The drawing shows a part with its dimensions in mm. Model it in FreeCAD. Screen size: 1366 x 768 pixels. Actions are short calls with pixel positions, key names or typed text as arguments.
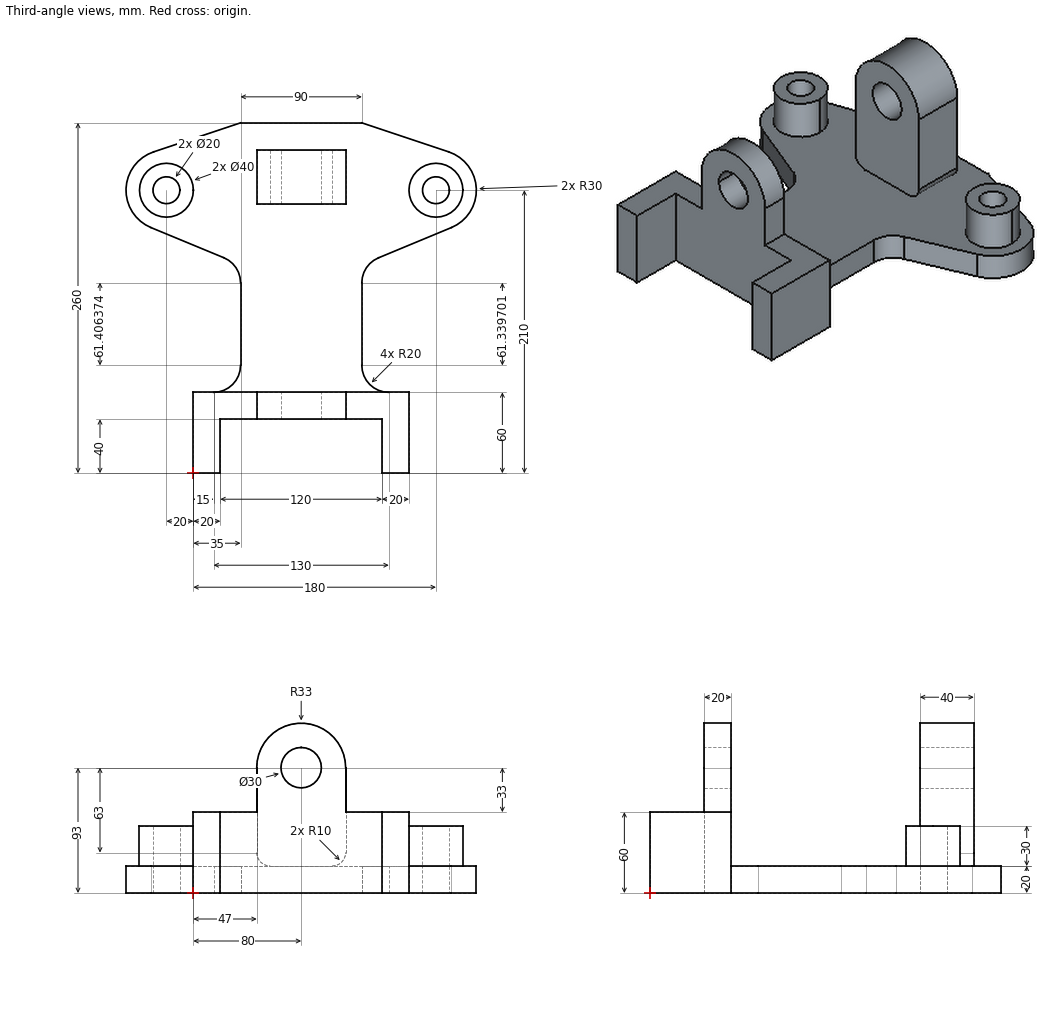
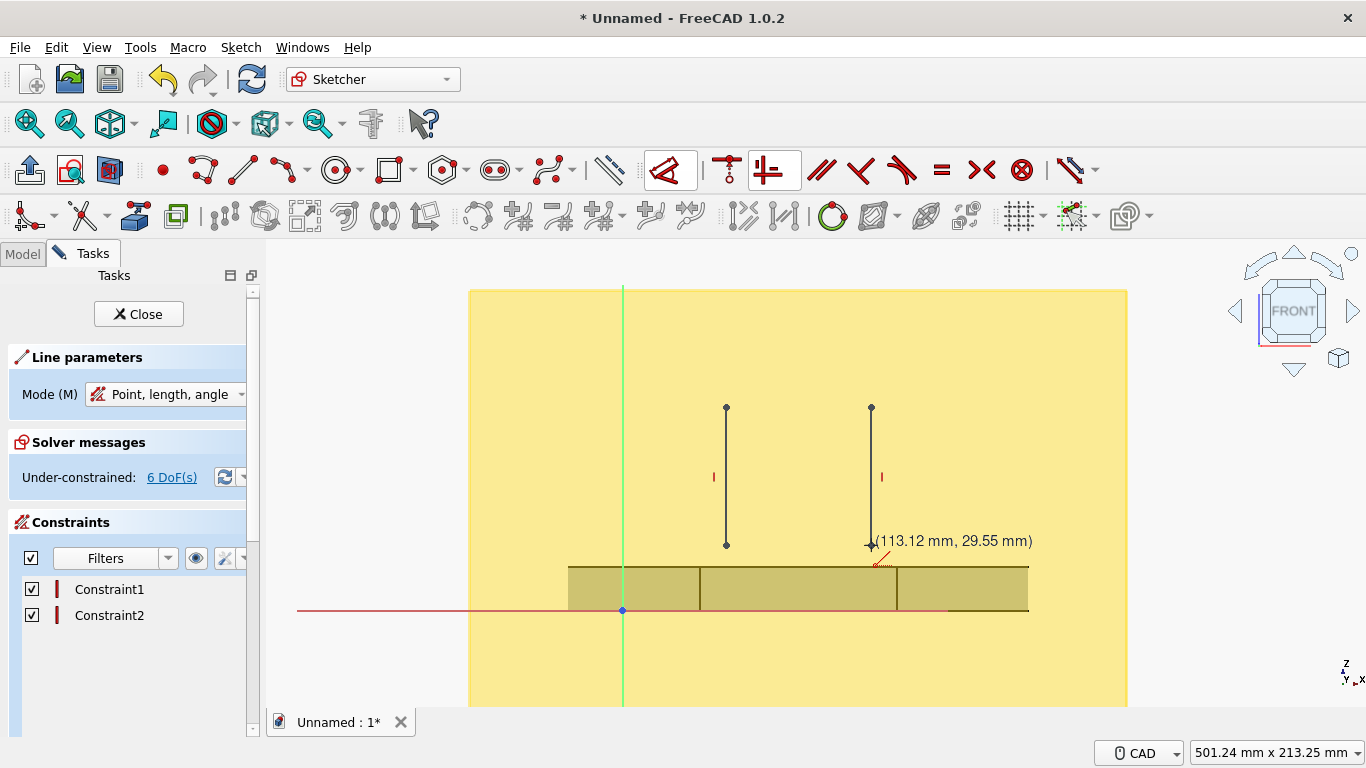
click(849, 567)
click(748, 567)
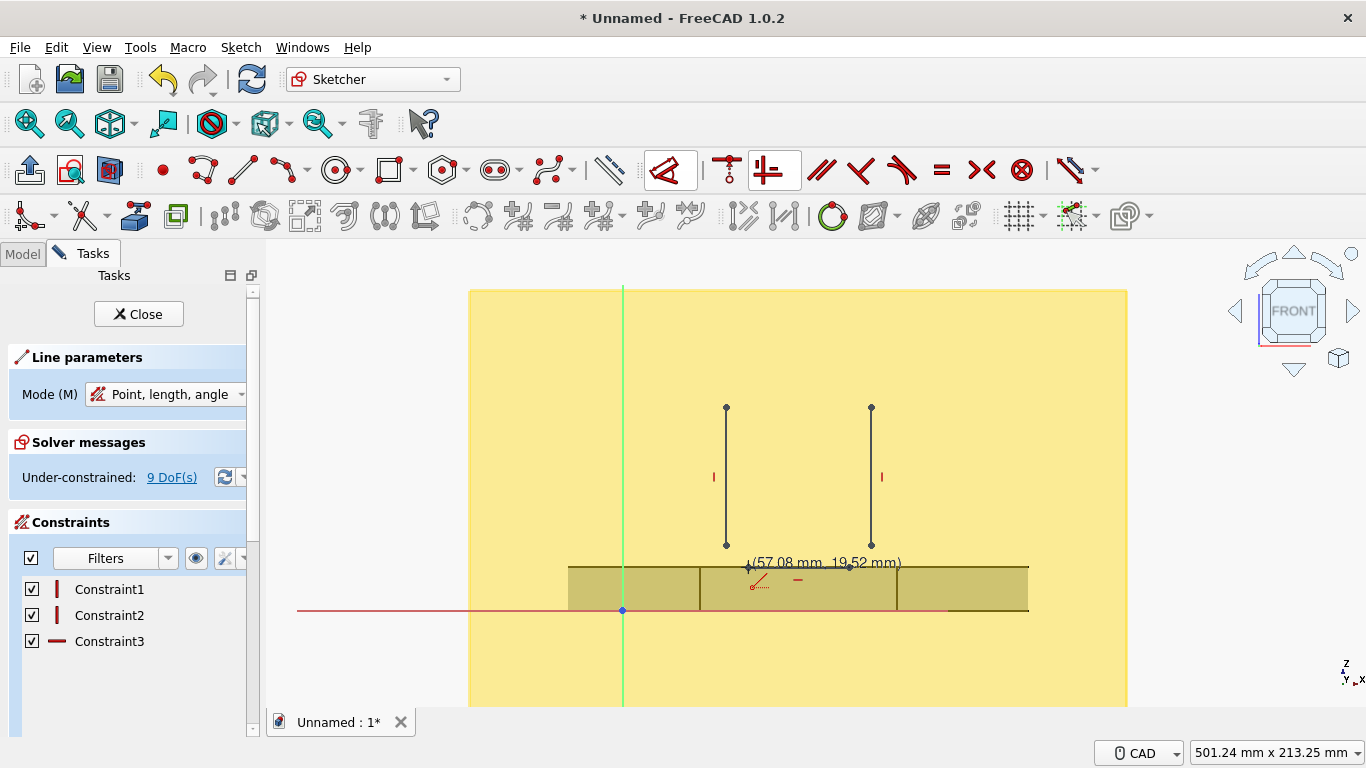
click(284, 170)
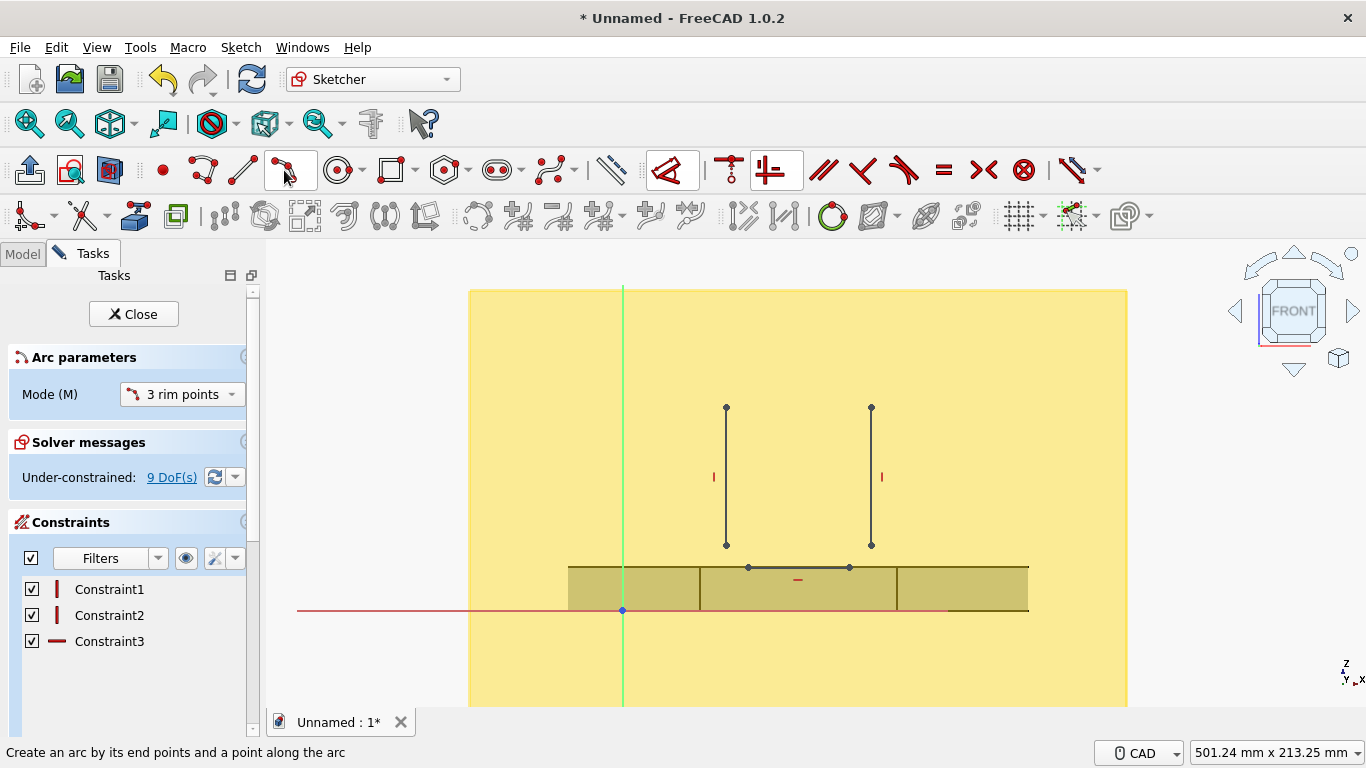
click(726, 408)
click(871, 408)
click(798, 334)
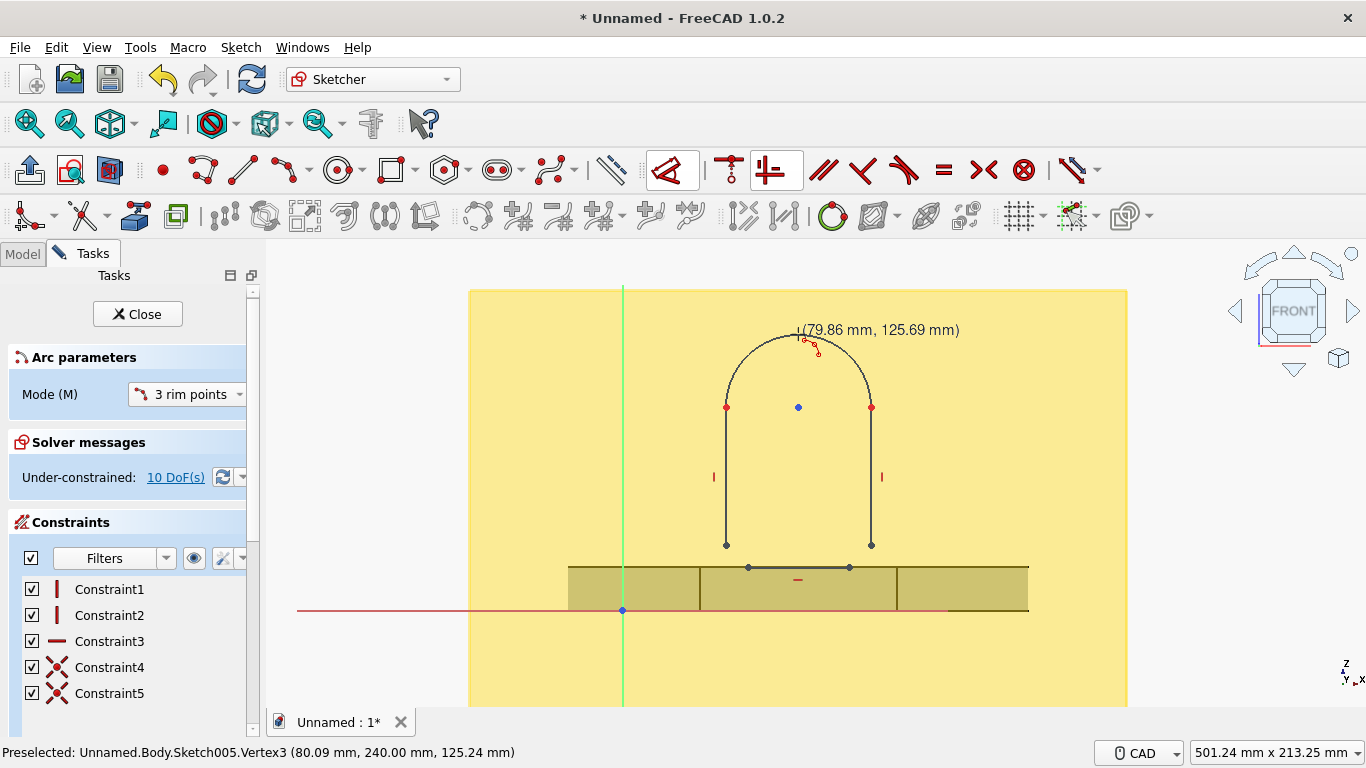
click(871, 546)
click(849, 568)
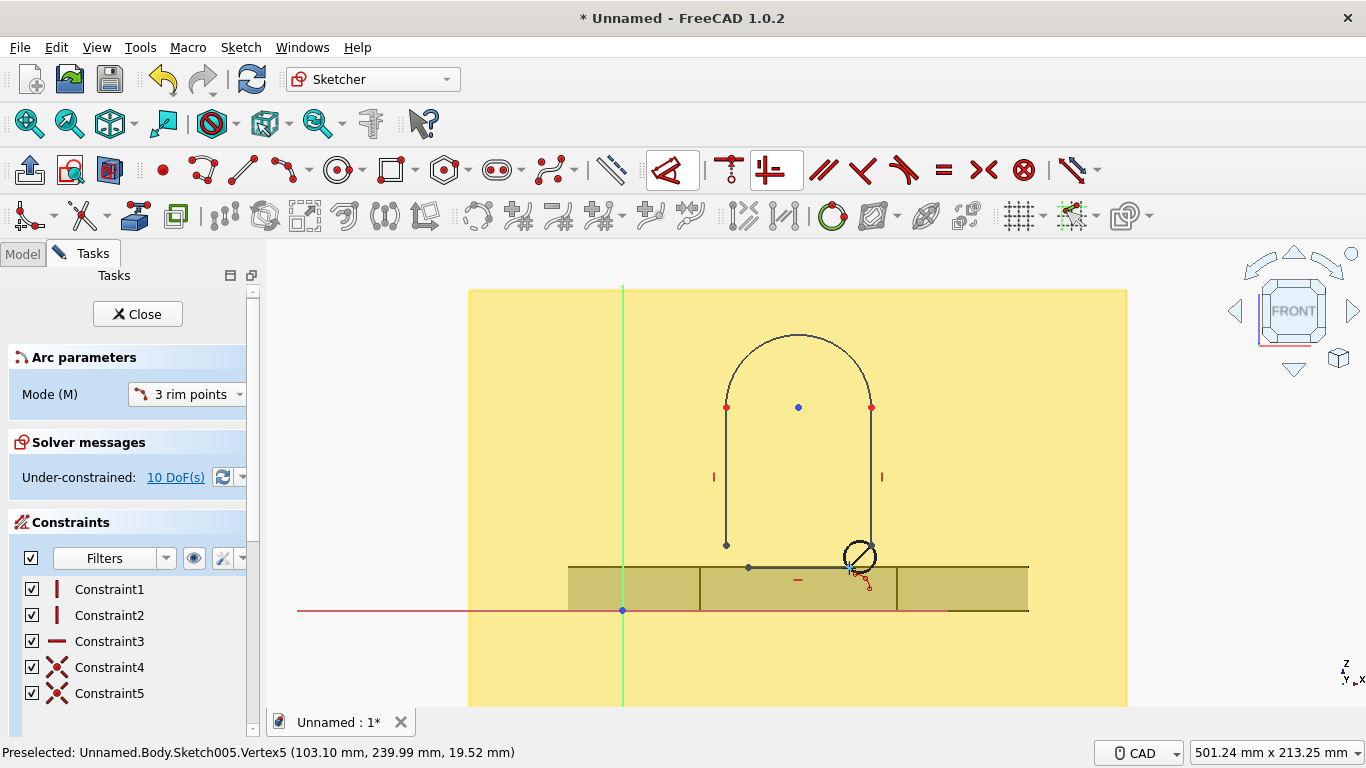
scroll(864, 561, up, 5)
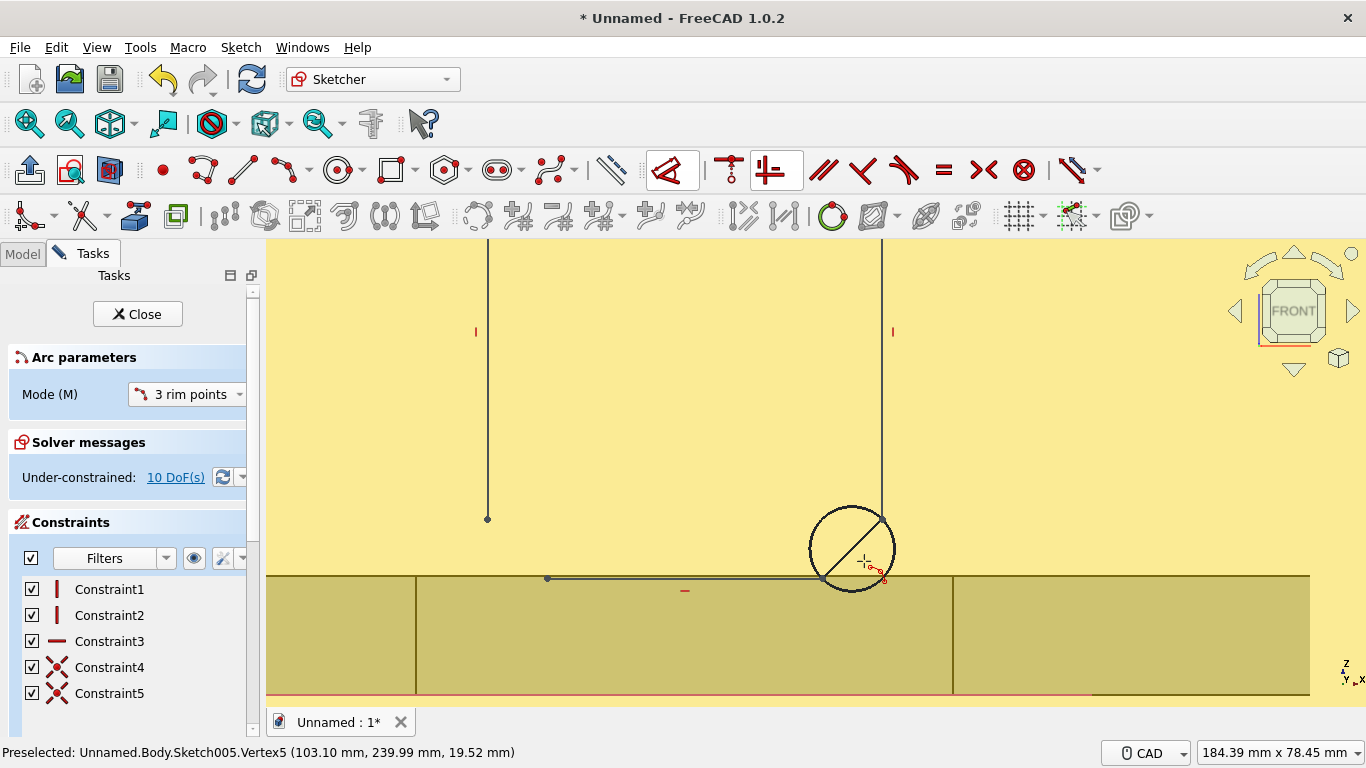
click(864, 559)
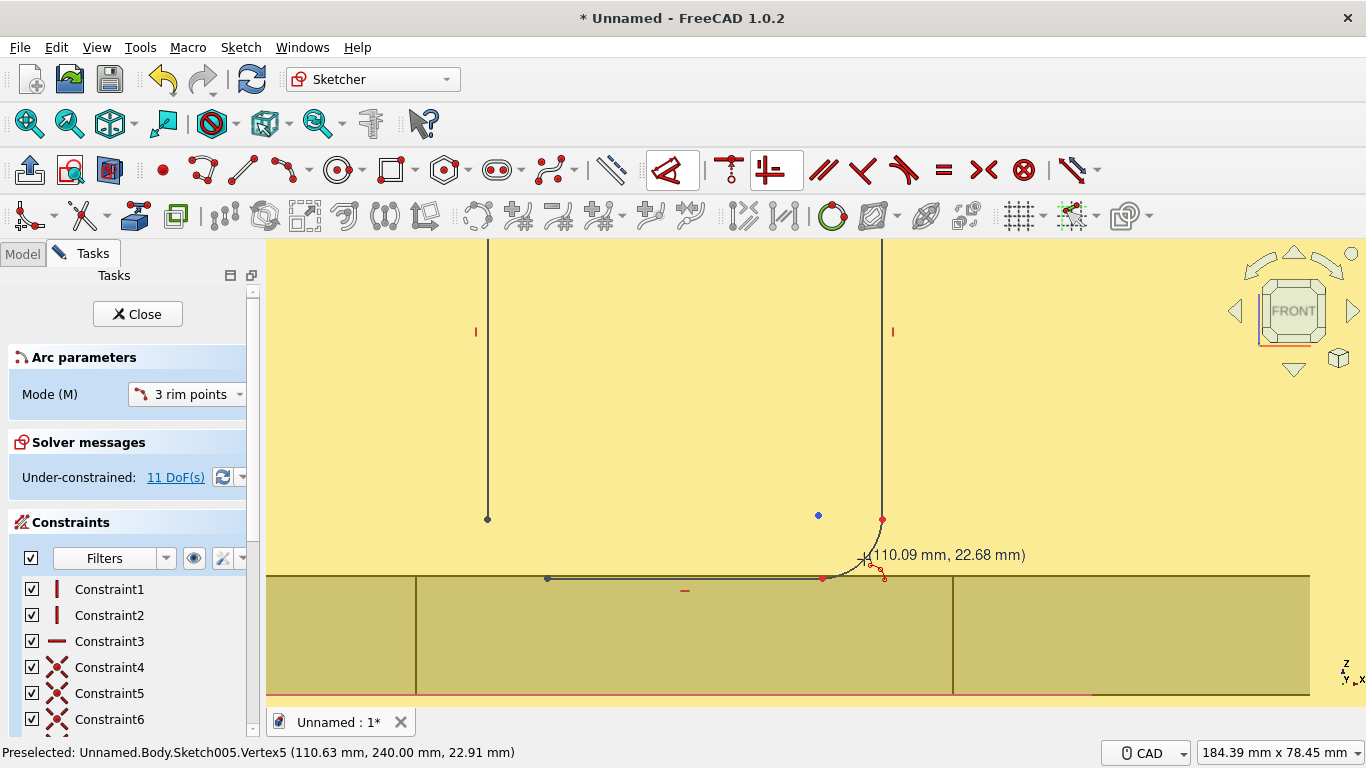
click(548, 579)
click(488, 519)
click(505, 559)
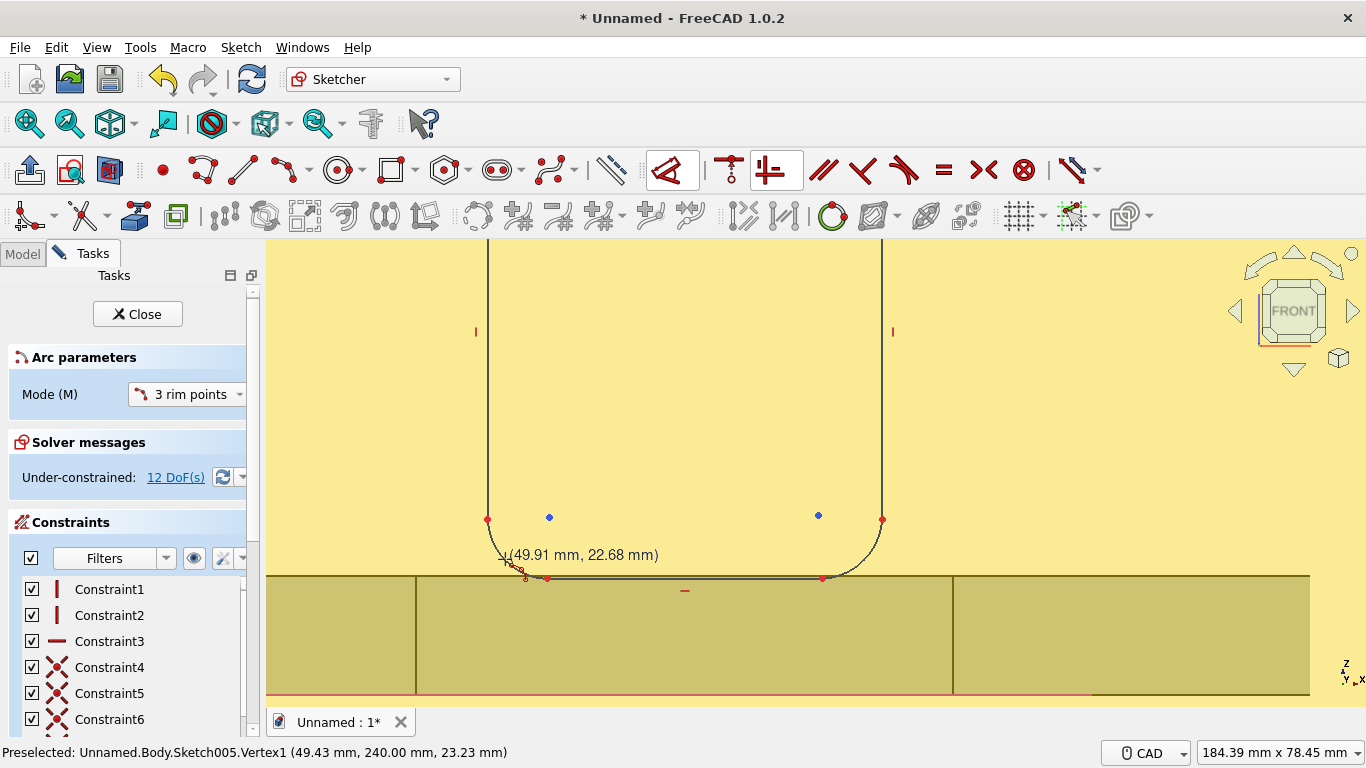
click(338, 170)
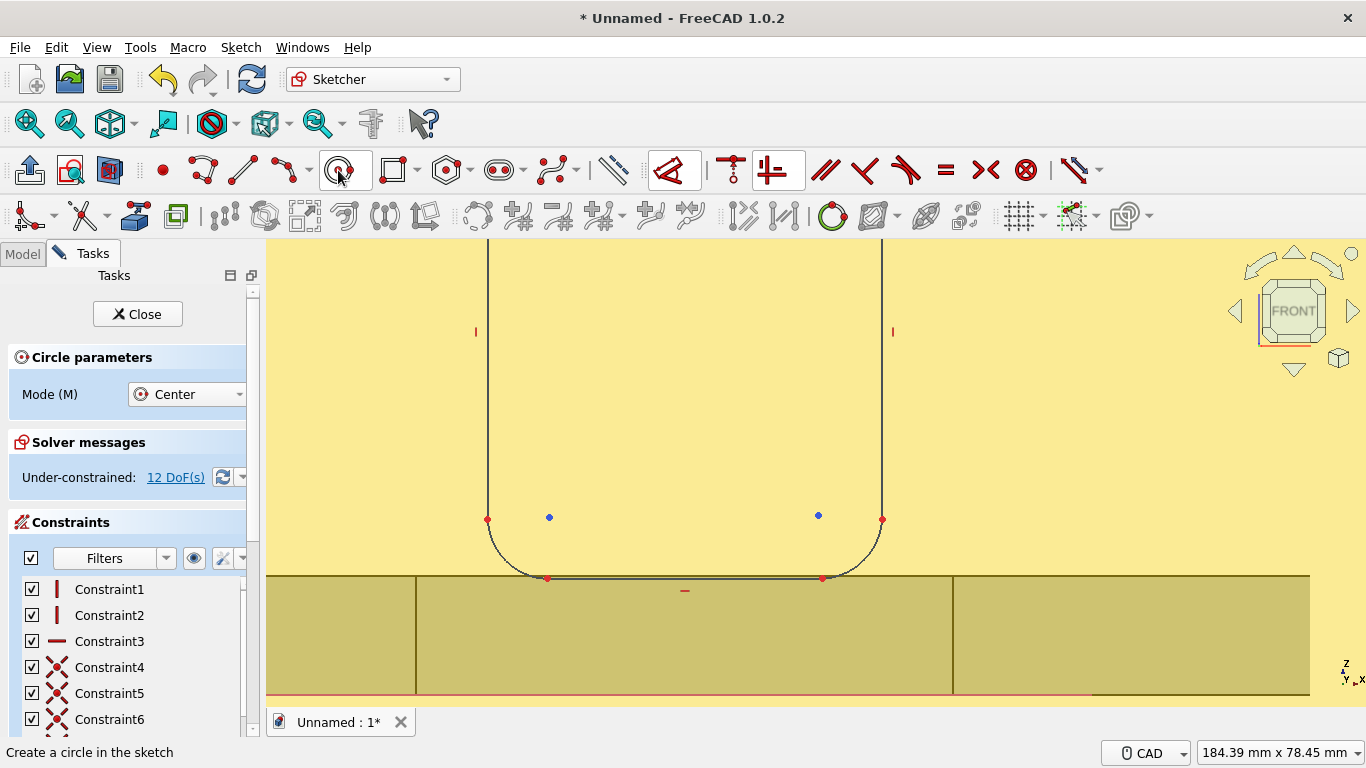
scroll(866, 562, down, 5)